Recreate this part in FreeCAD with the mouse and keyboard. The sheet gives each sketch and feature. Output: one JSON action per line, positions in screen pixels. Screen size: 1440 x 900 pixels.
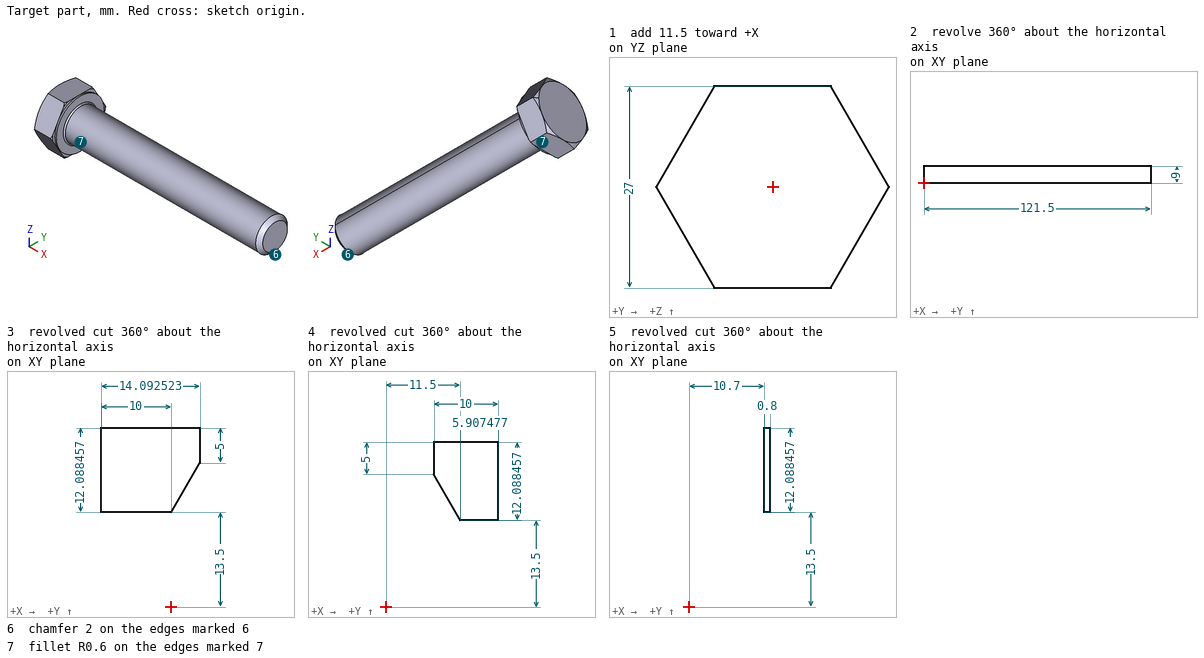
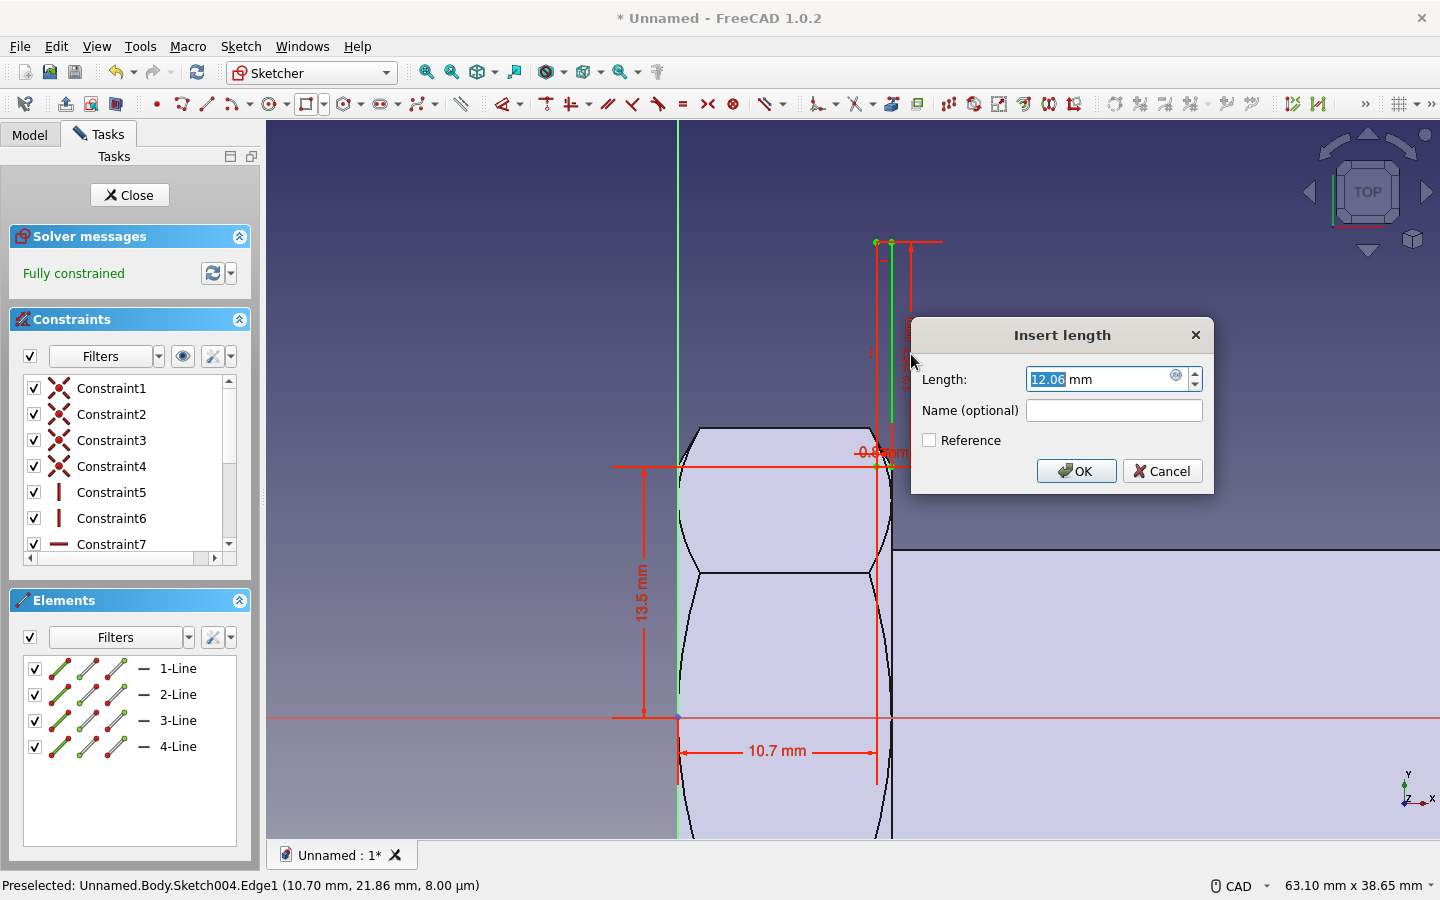
{"action": "type", "text": "12.088457"}
{"action": "key", "text": "Return"}
{"action": "key", "text": "Escape"}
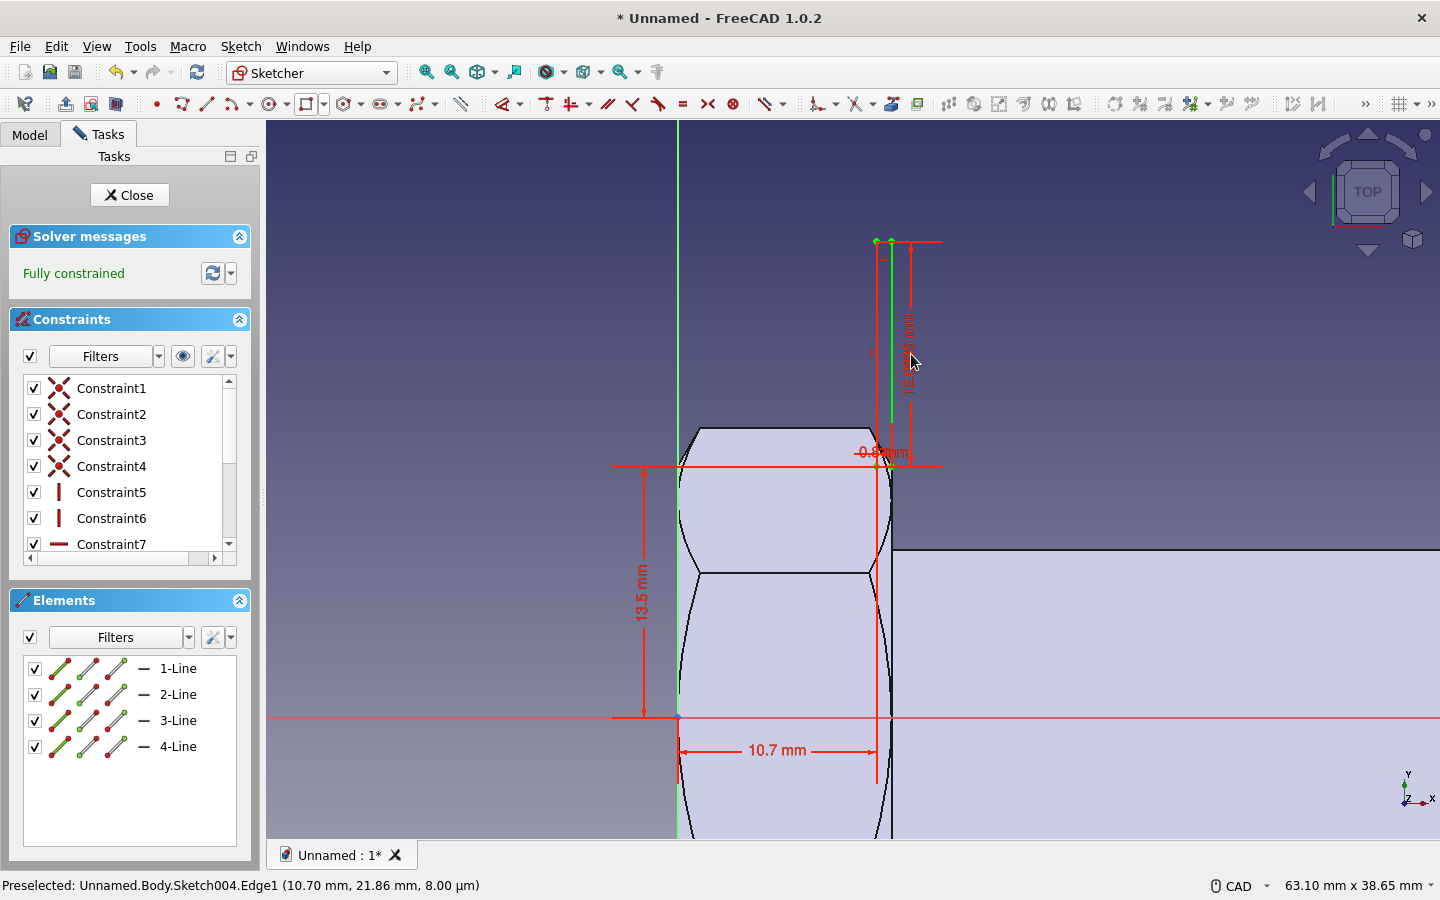
{"action": "left_click", "coordinate": [130, 195]}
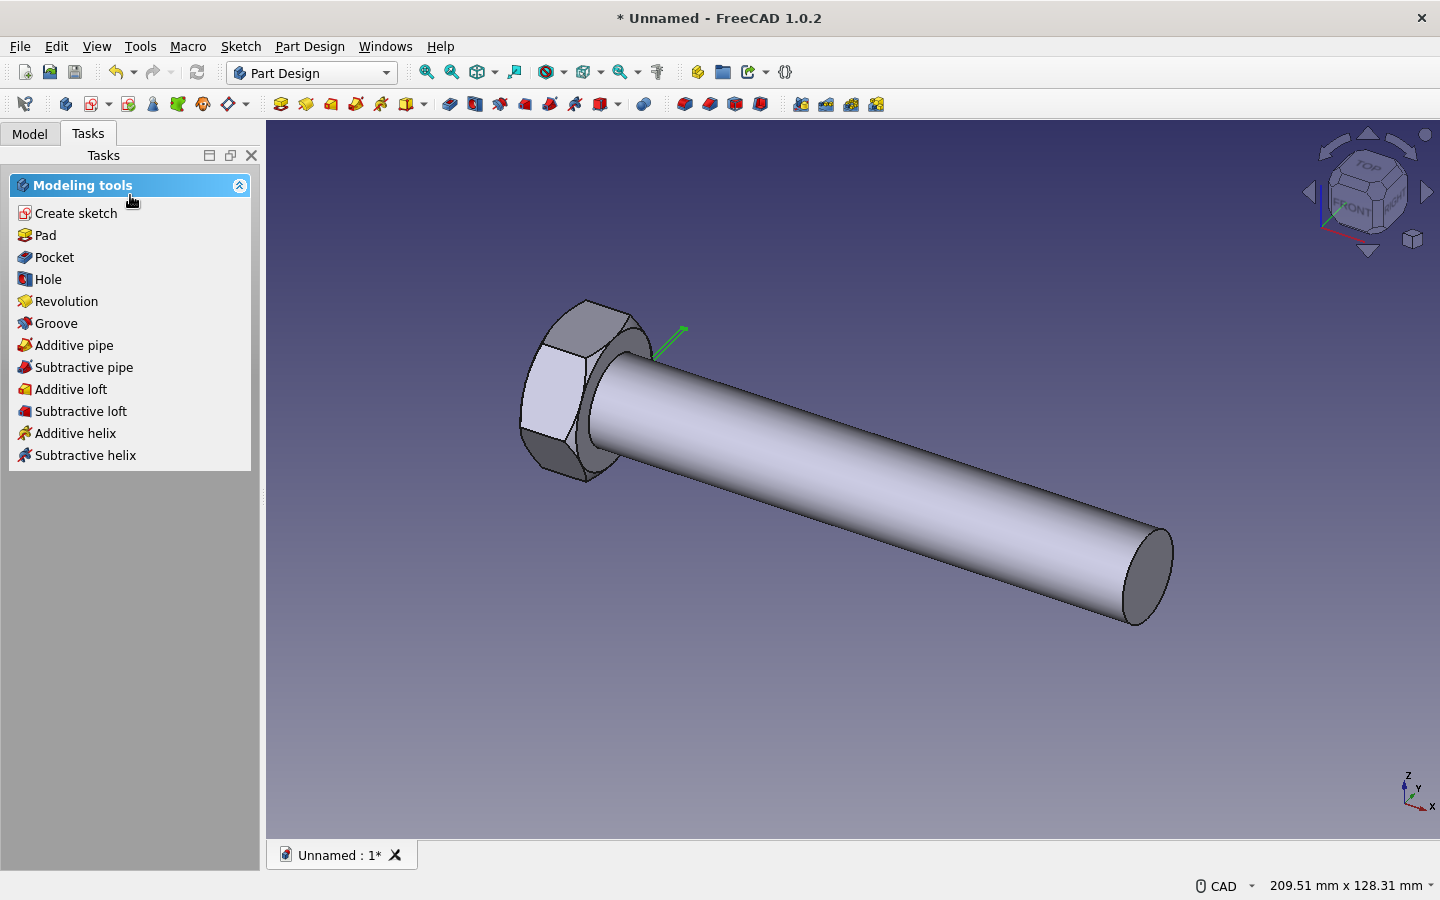
{"action": "left_click", "coordinate": [500, 104]}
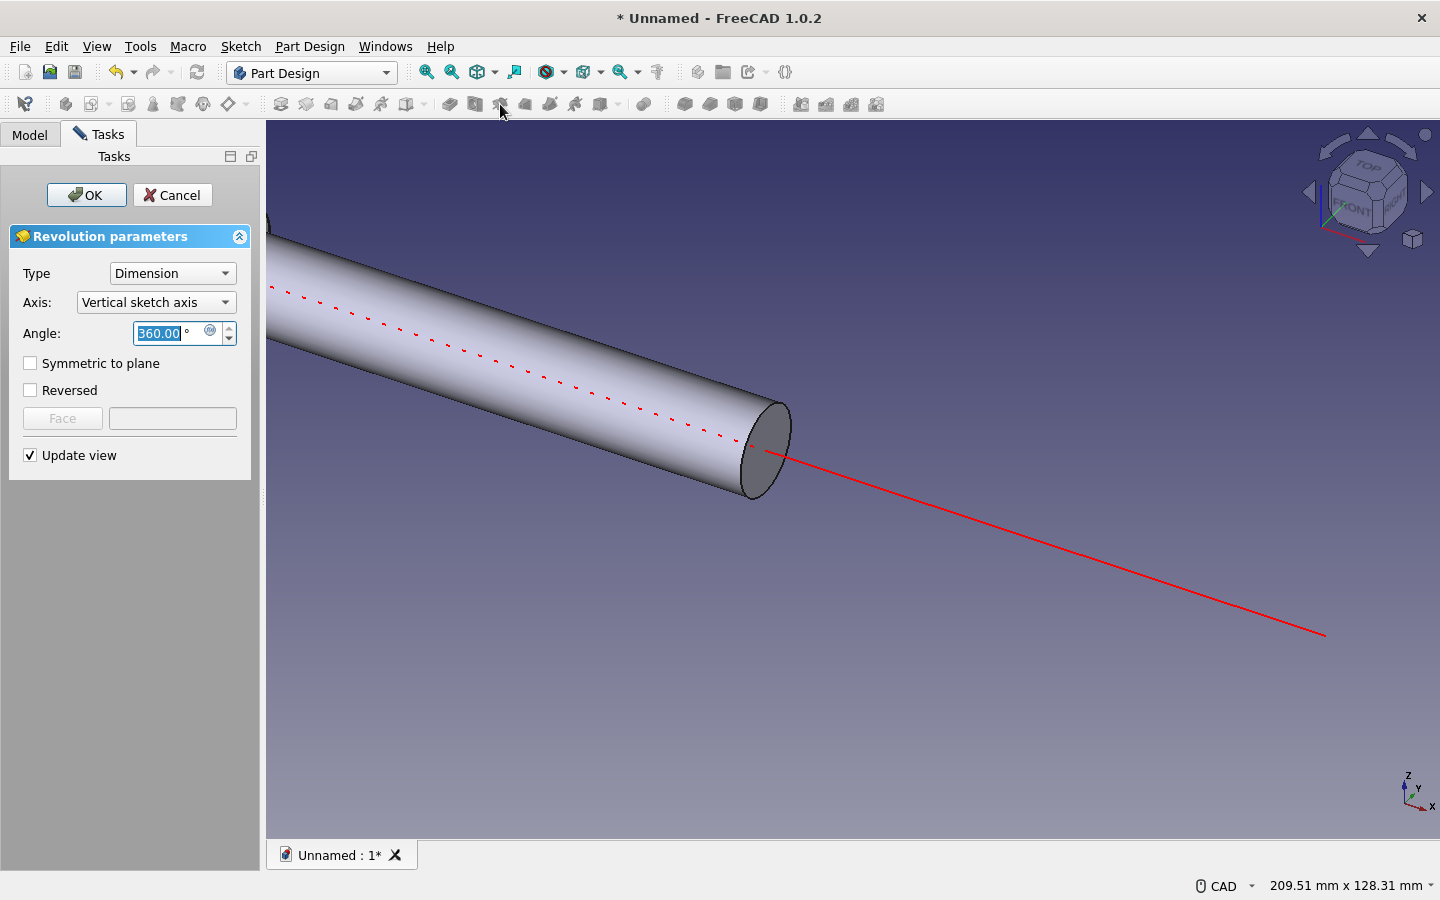
{"action": "left_click", "coordinate": [157, 302]}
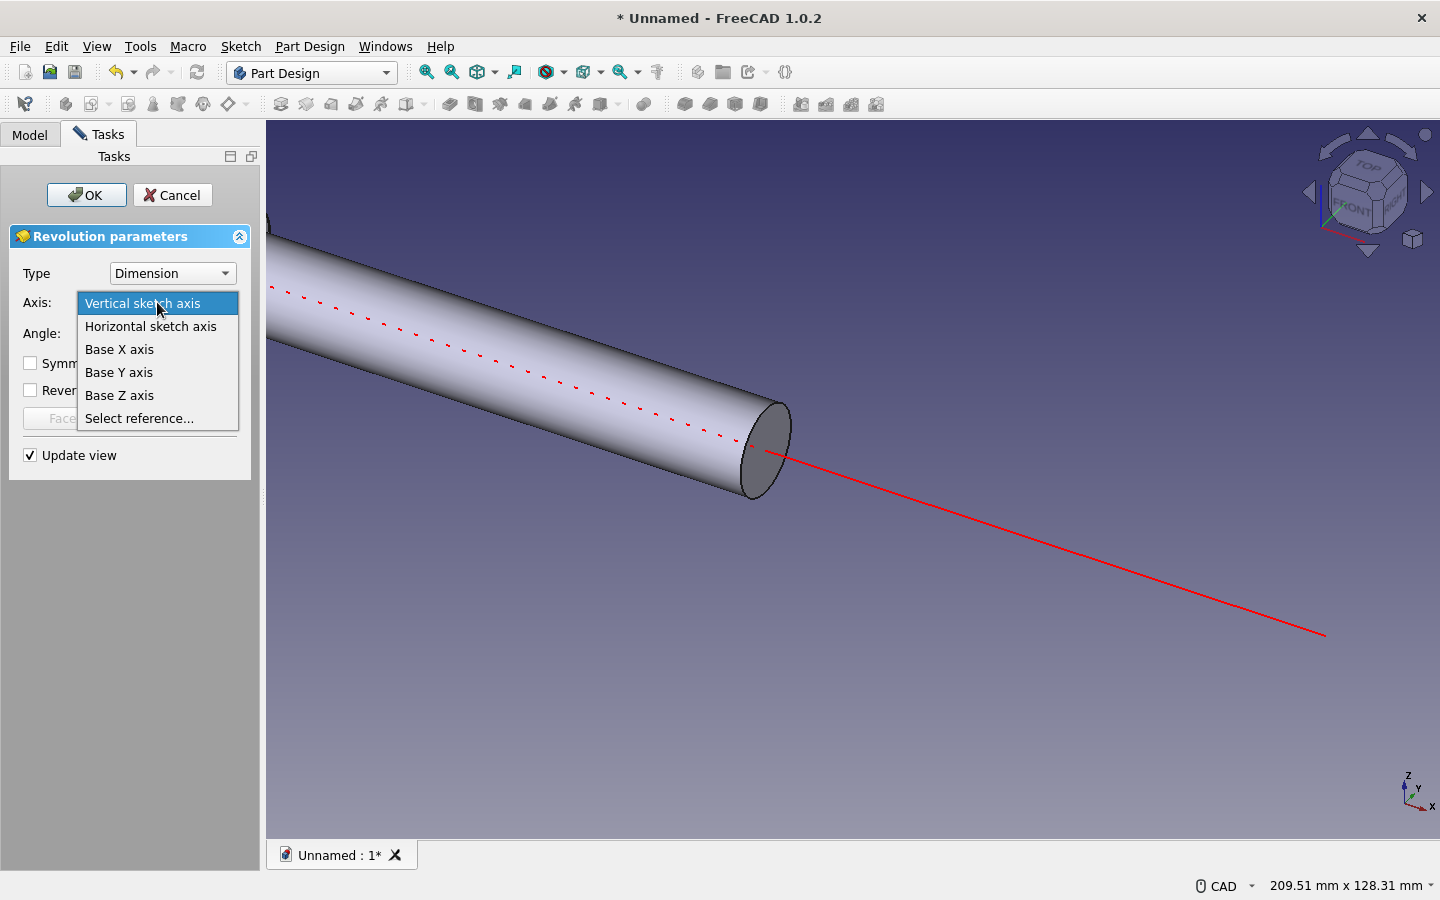
{"action": "left_click", "coordinate": [156, 326]}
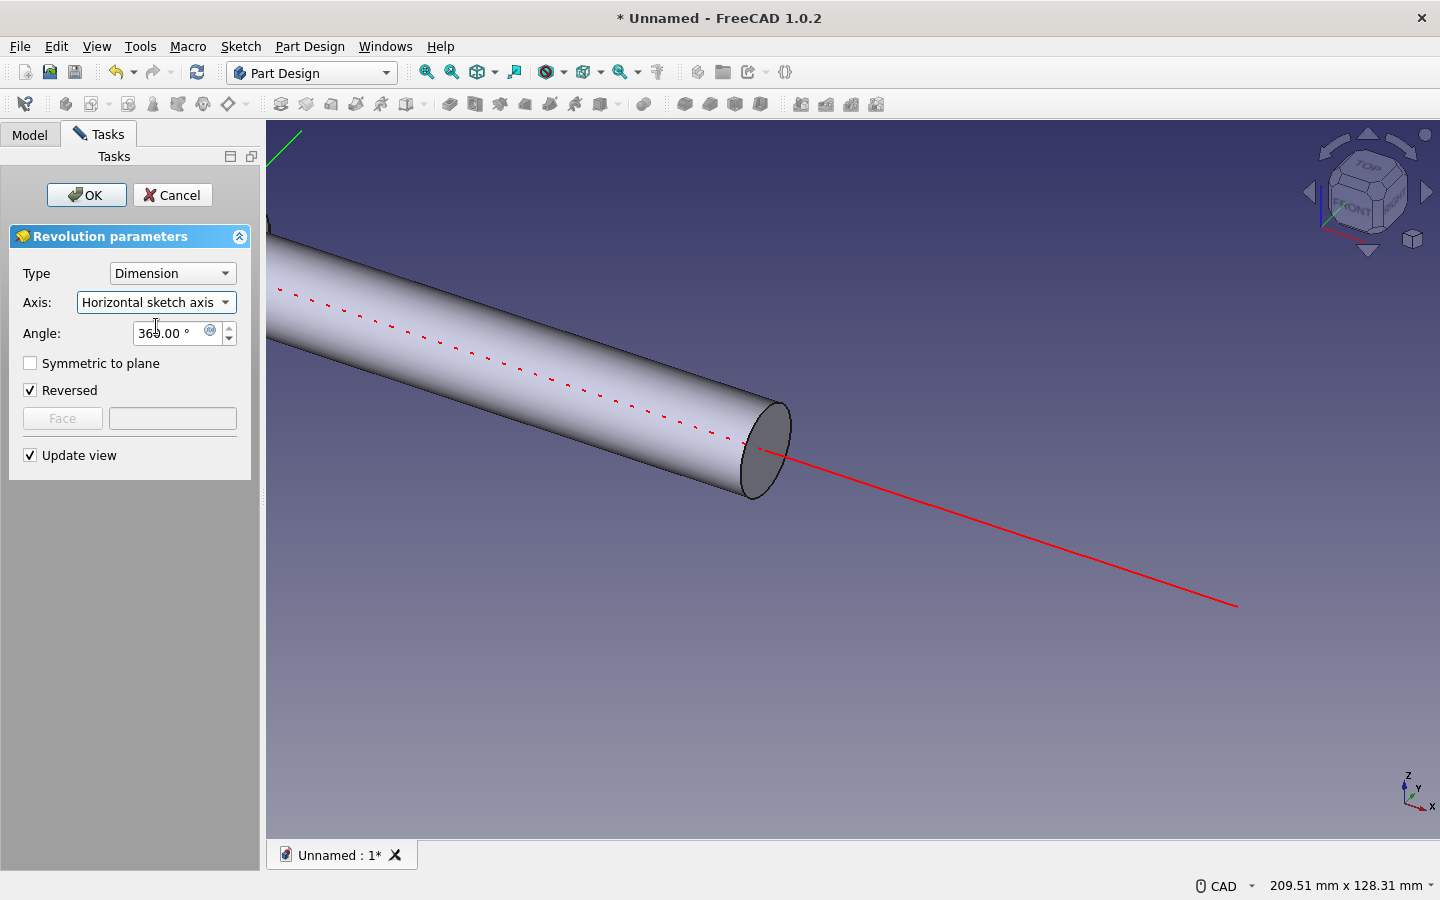
{"action": "left_click", "coordinate": [87, 195]}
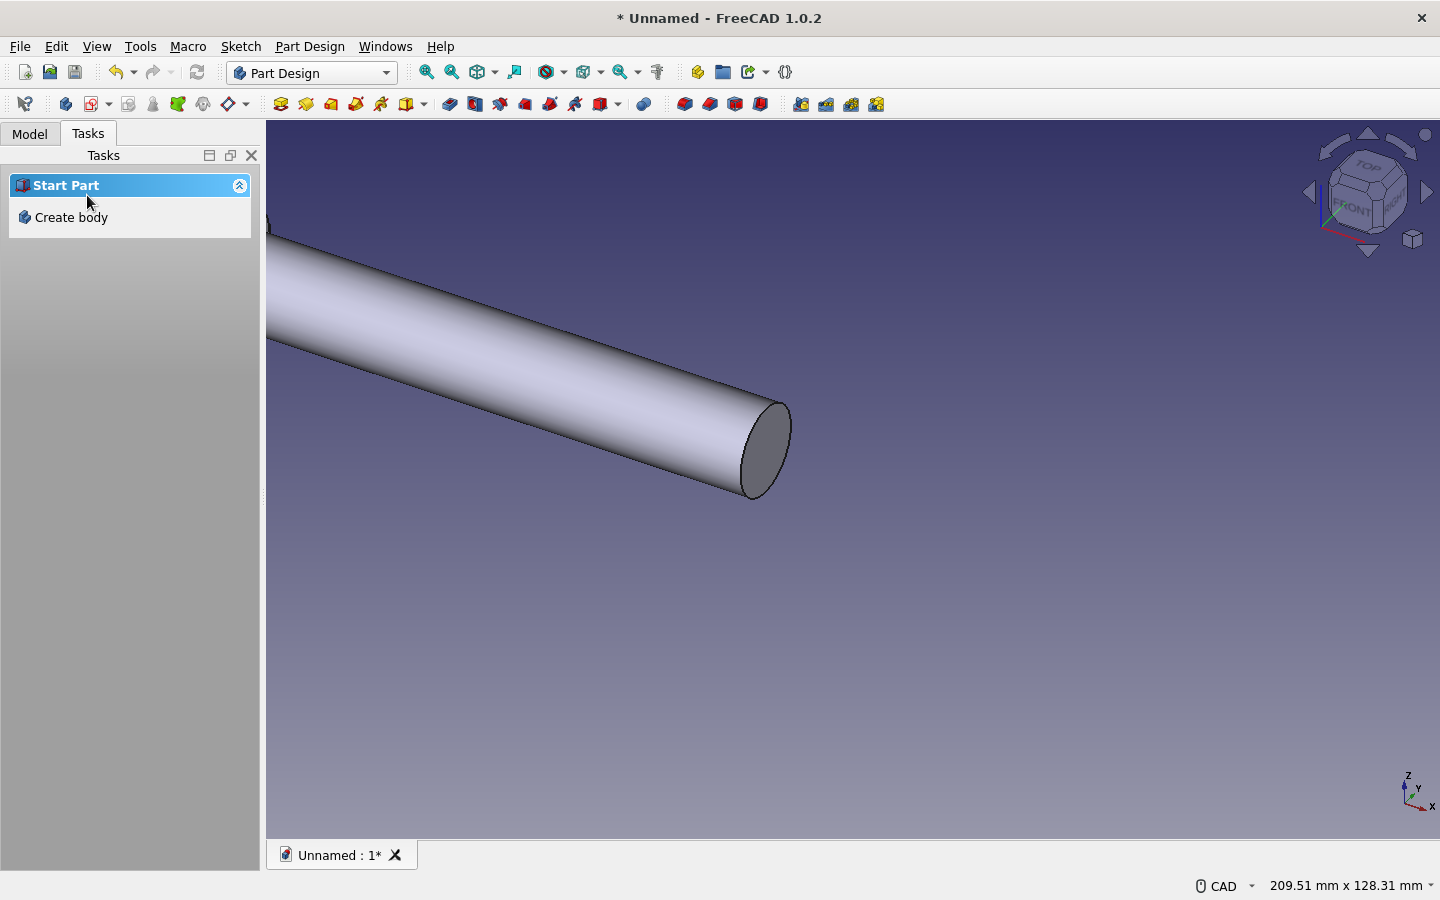
{"action": "left_click", "coordinate": [427, 72]}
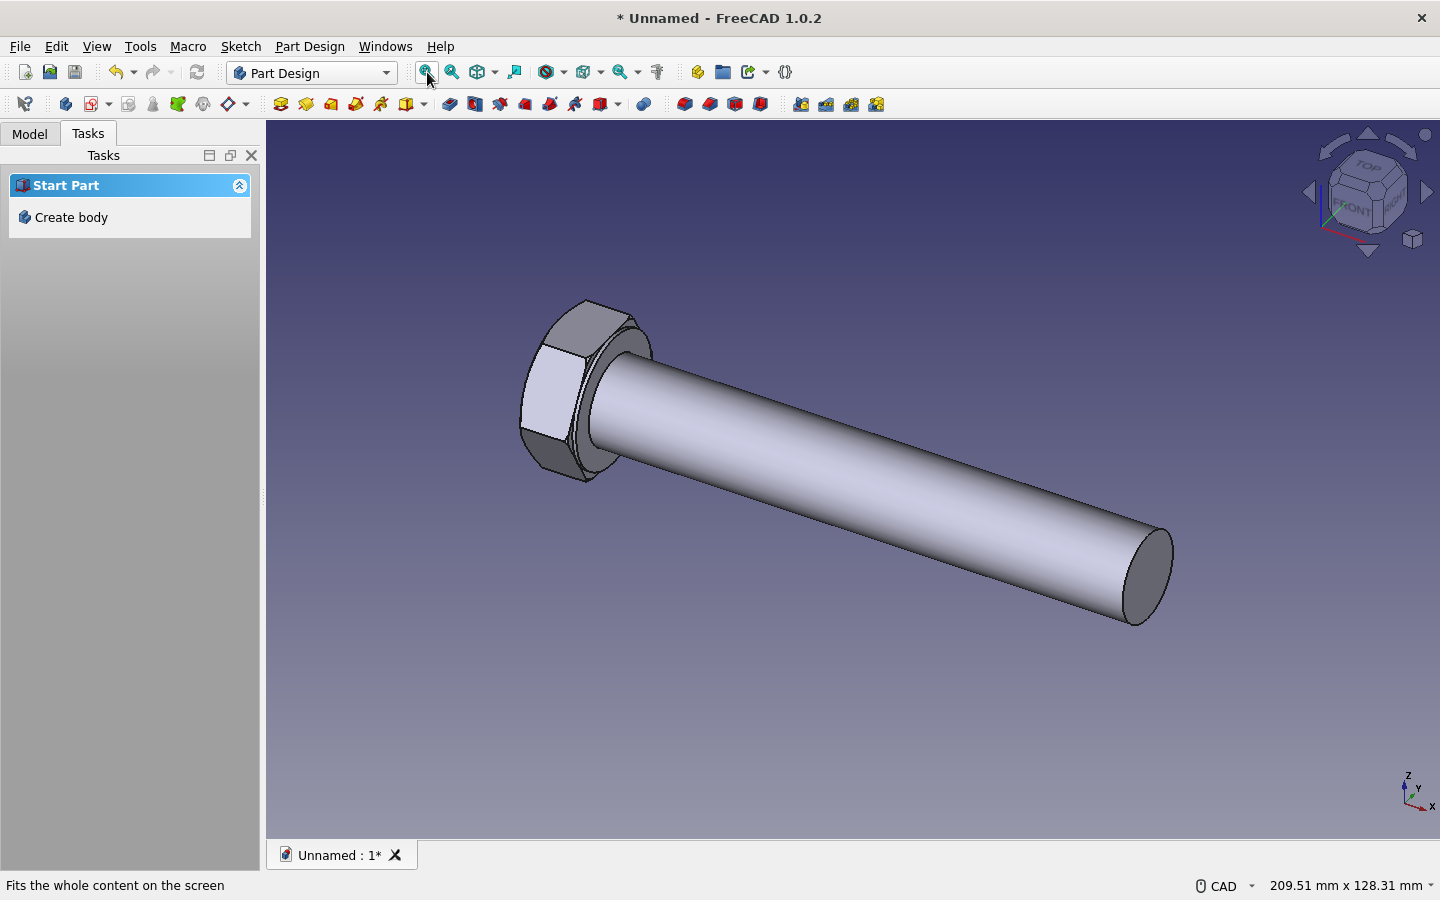
{"action": "left_click", "coordinate": [1123, 601]}